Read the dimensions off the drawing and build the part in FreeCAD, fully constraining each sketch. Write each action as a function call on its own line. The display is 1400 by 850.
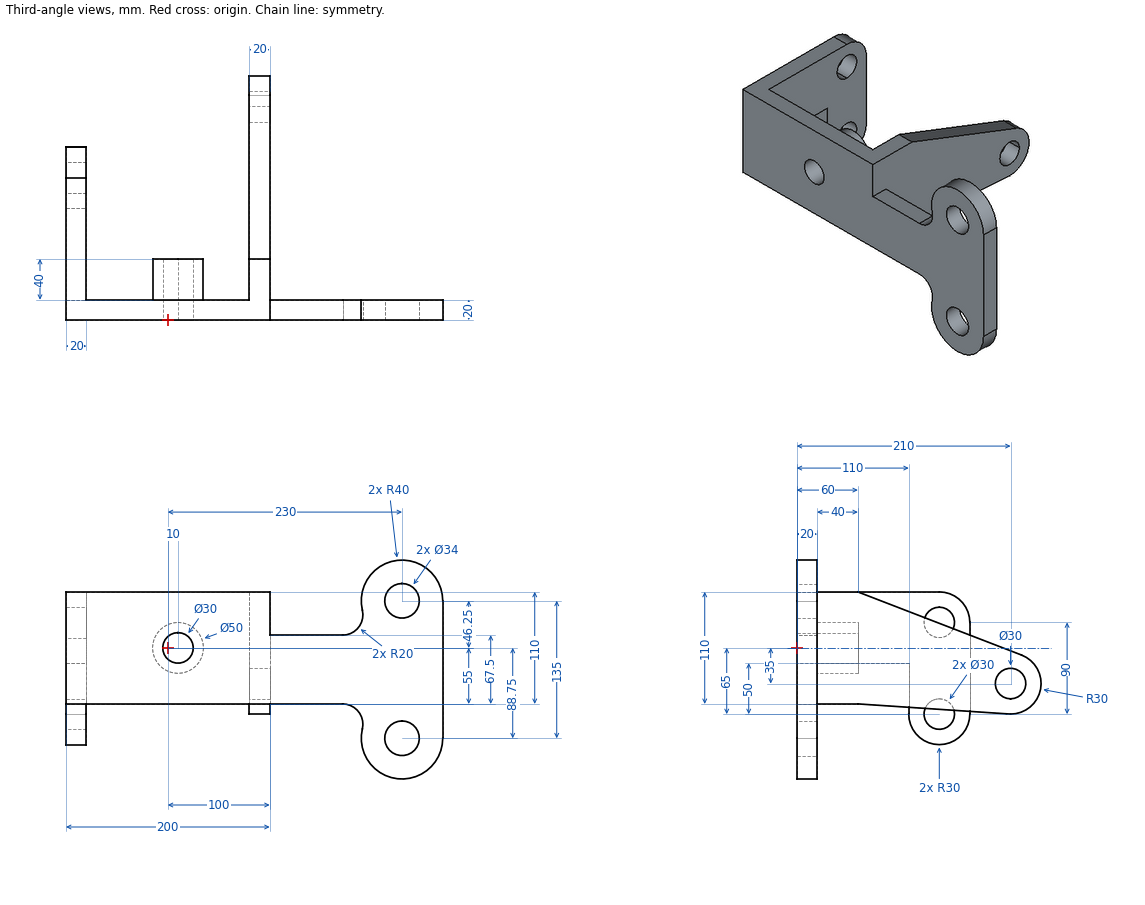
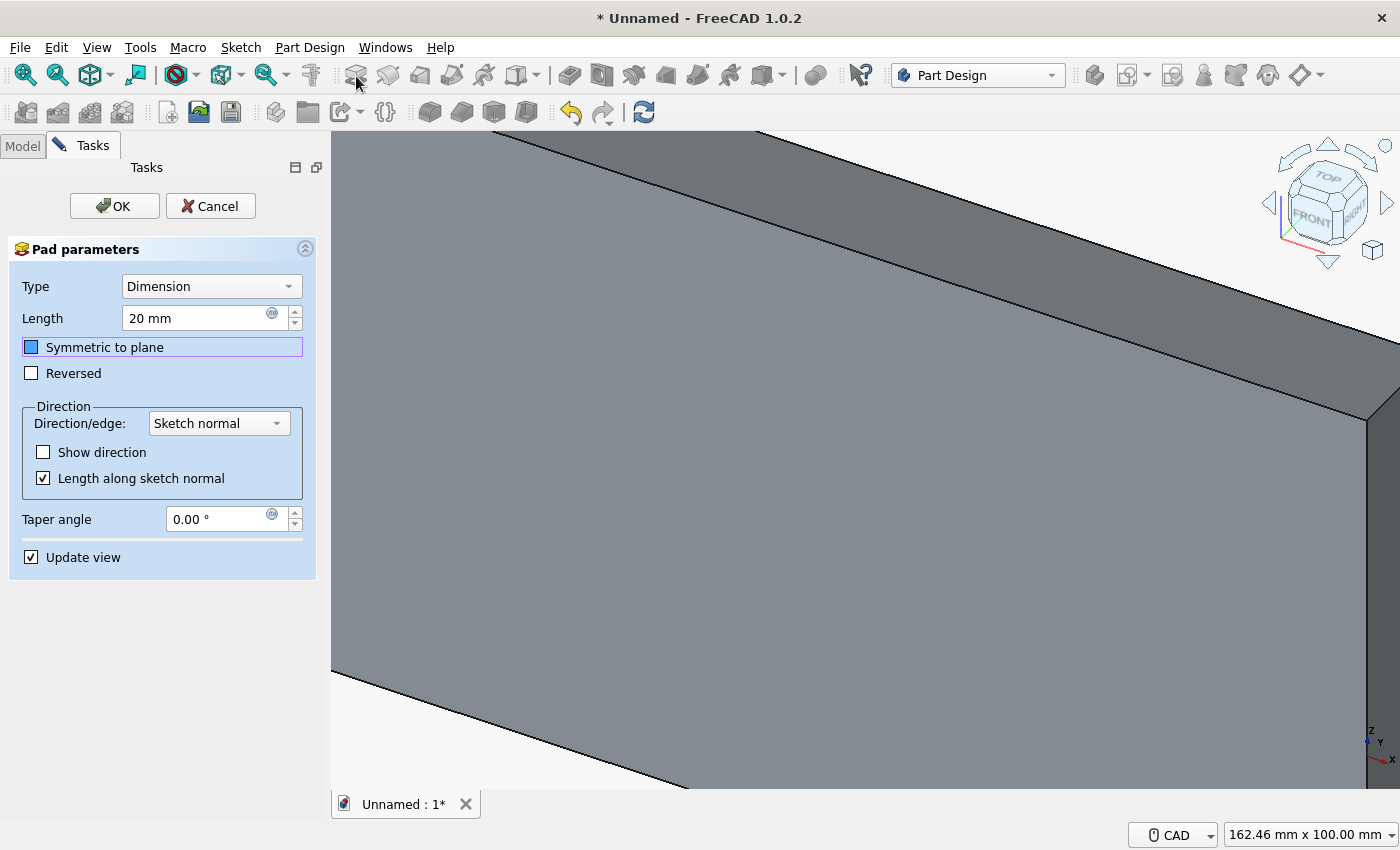
click(30, 373)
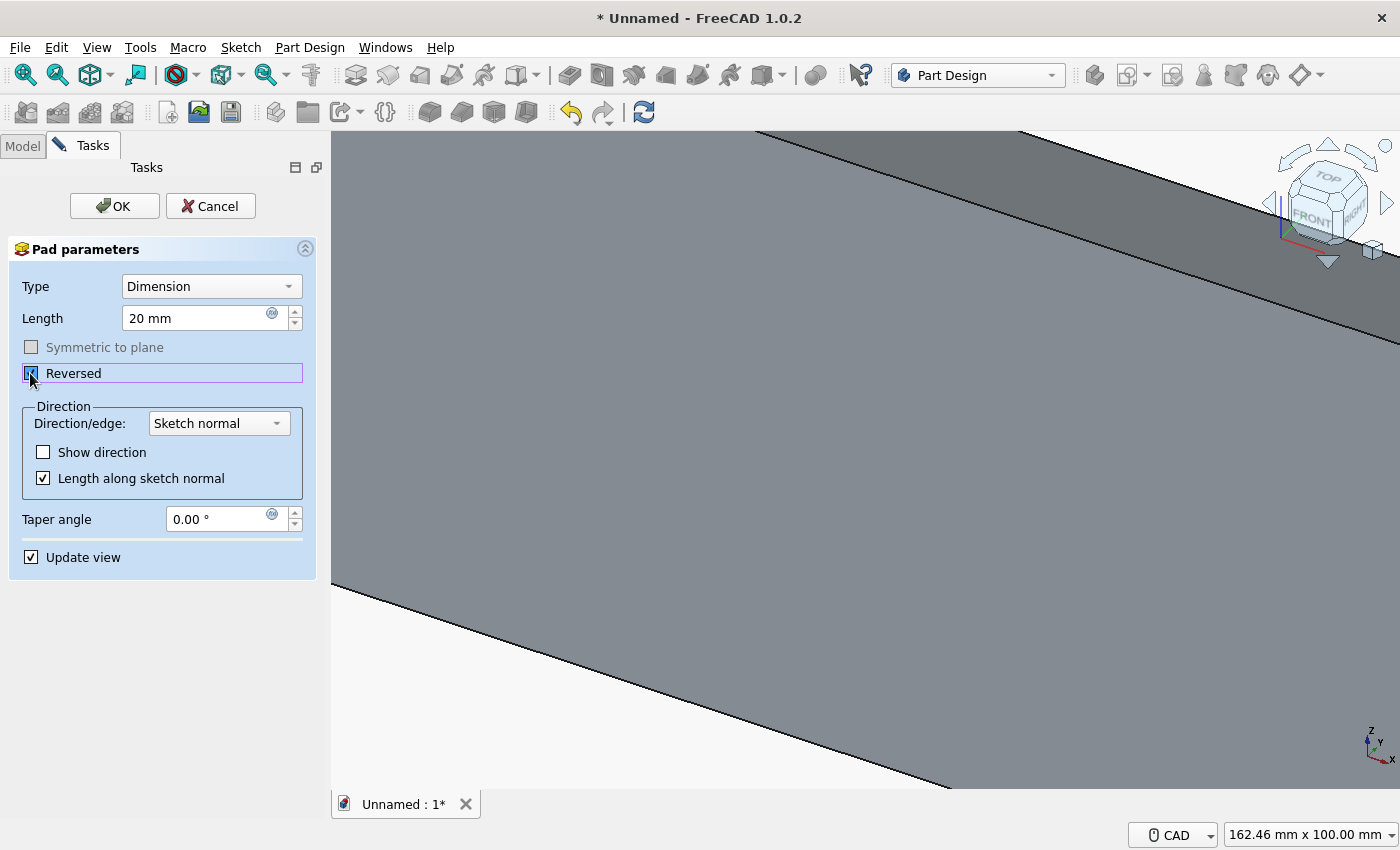
click(115, 206)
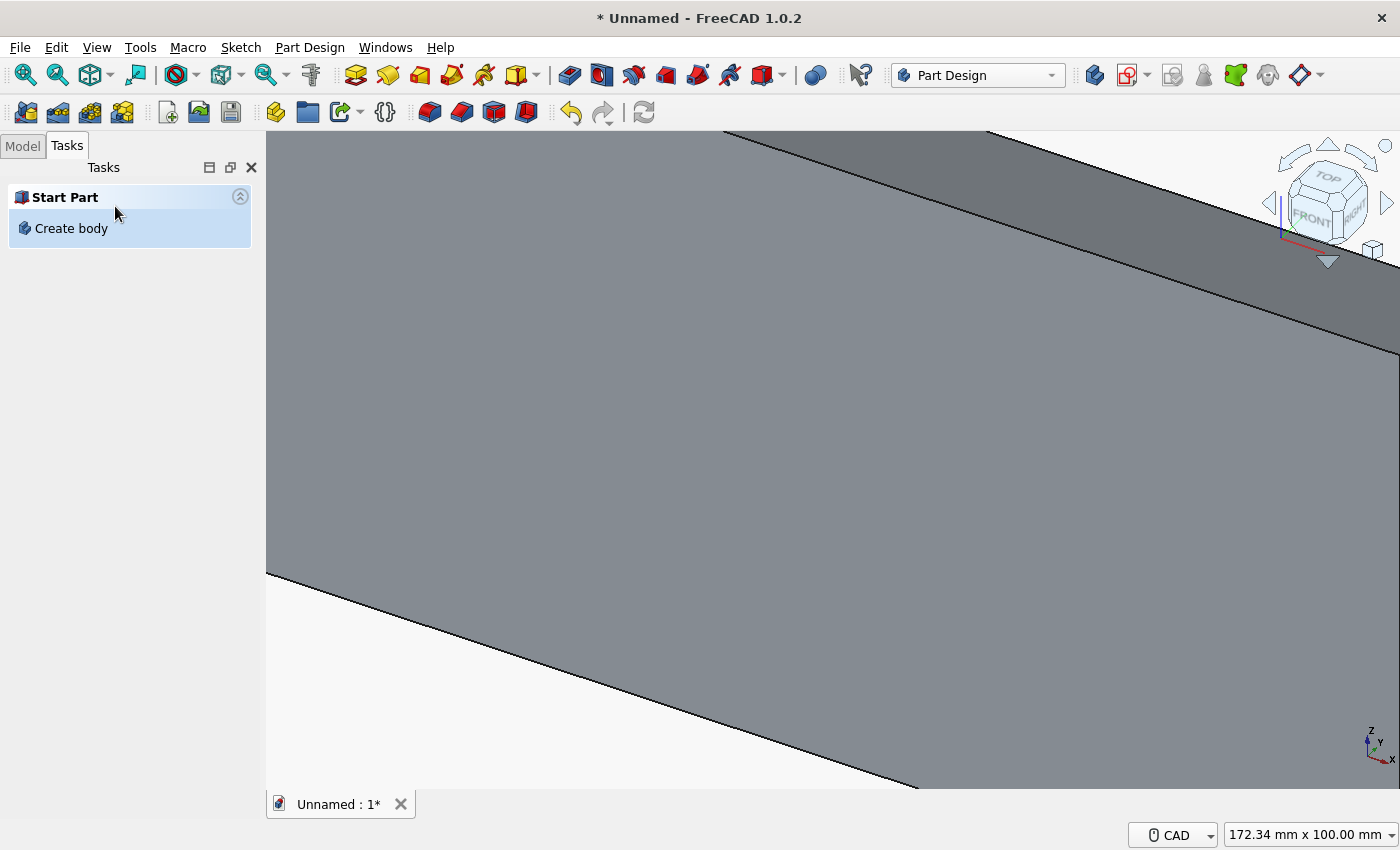
key(v)
key(f)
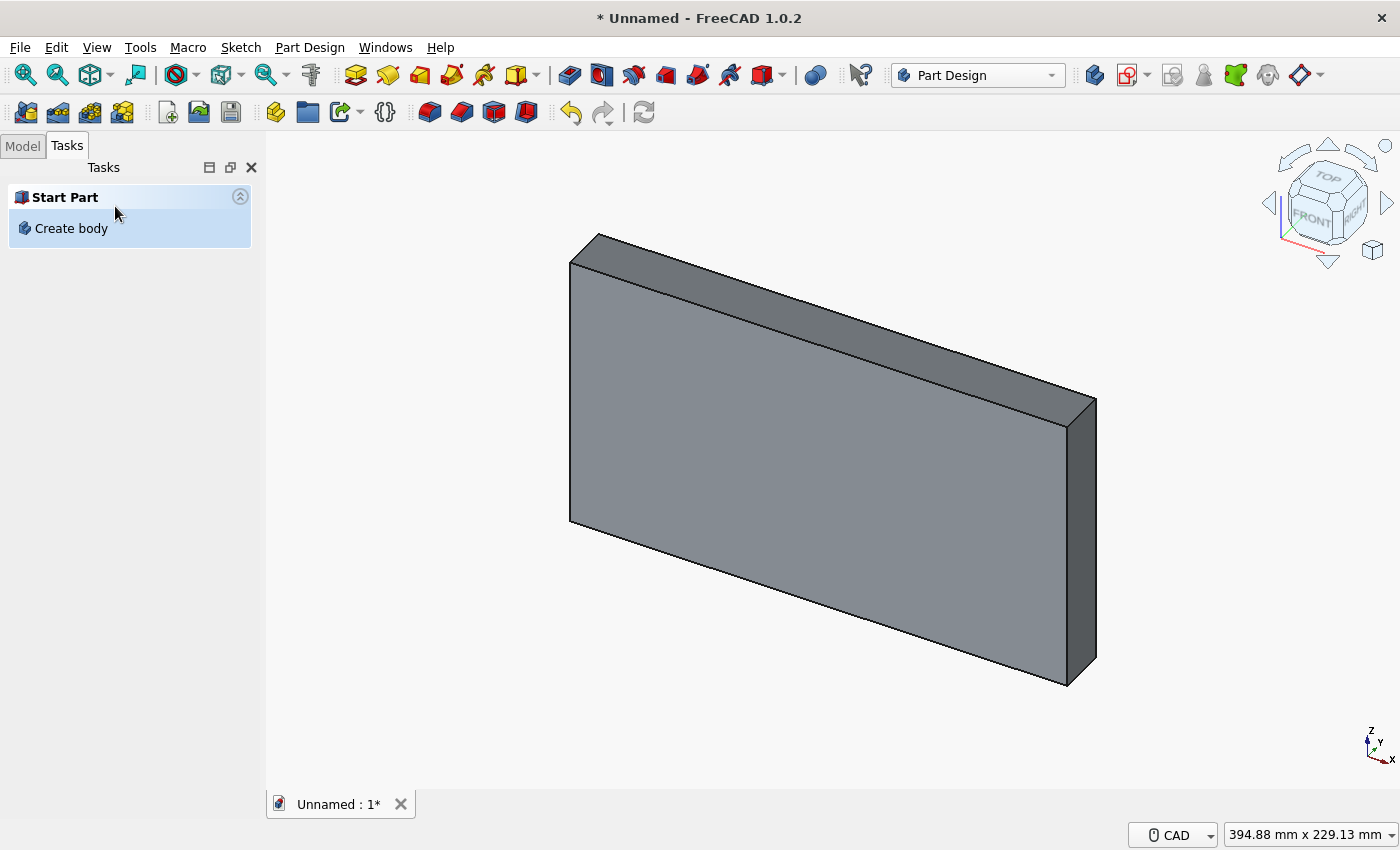
key(4)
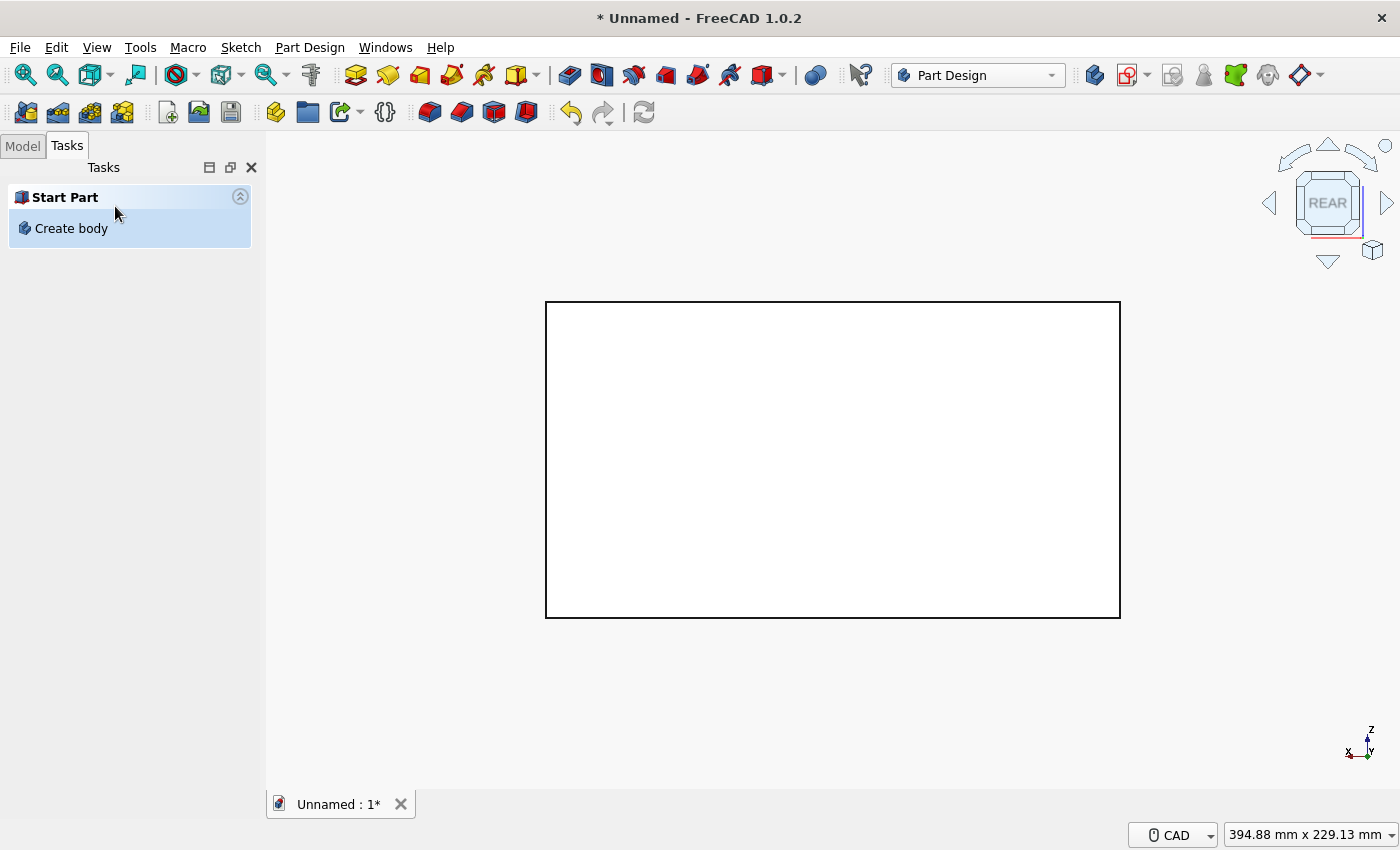
click(751, 459)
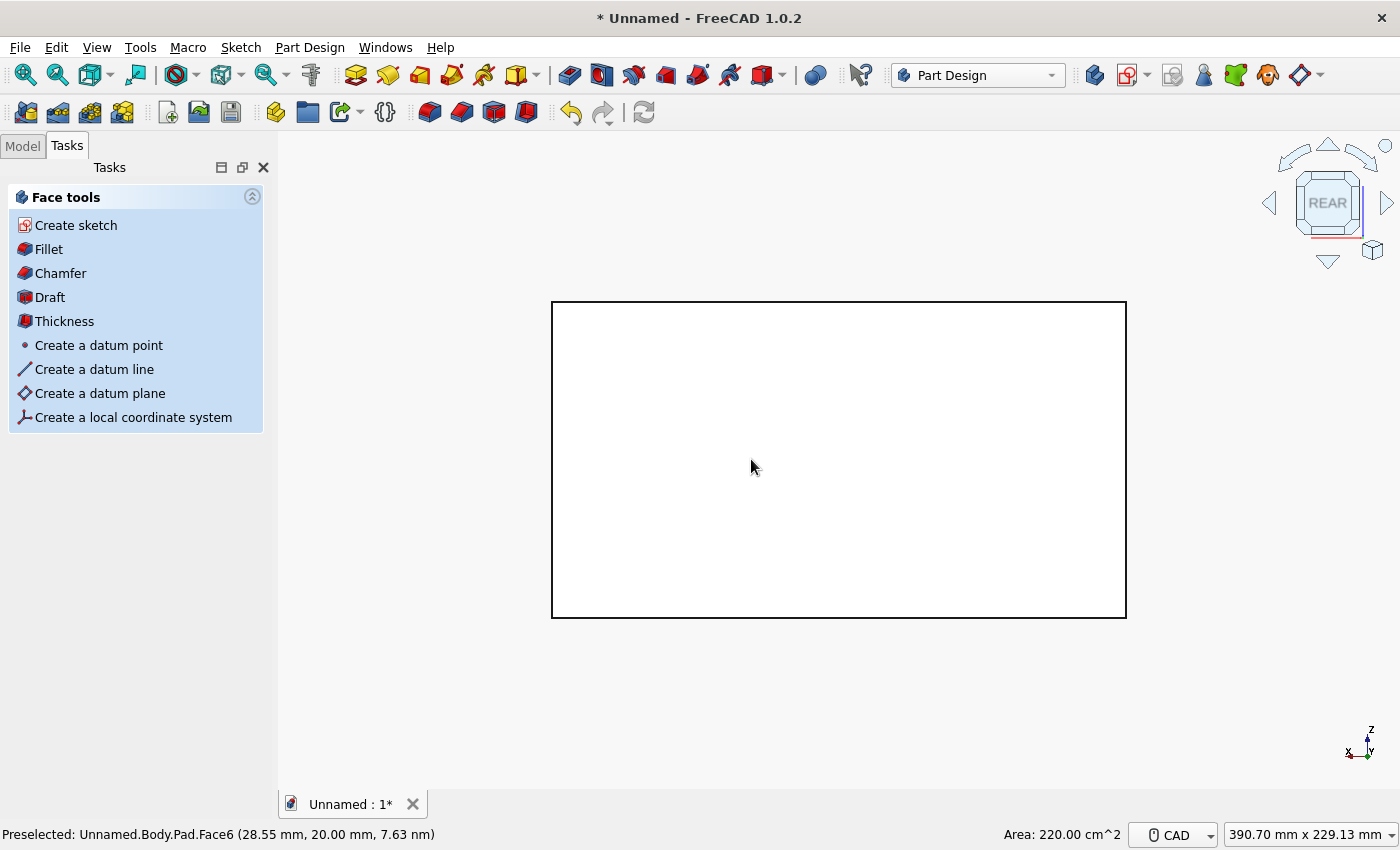
click(1128, 76)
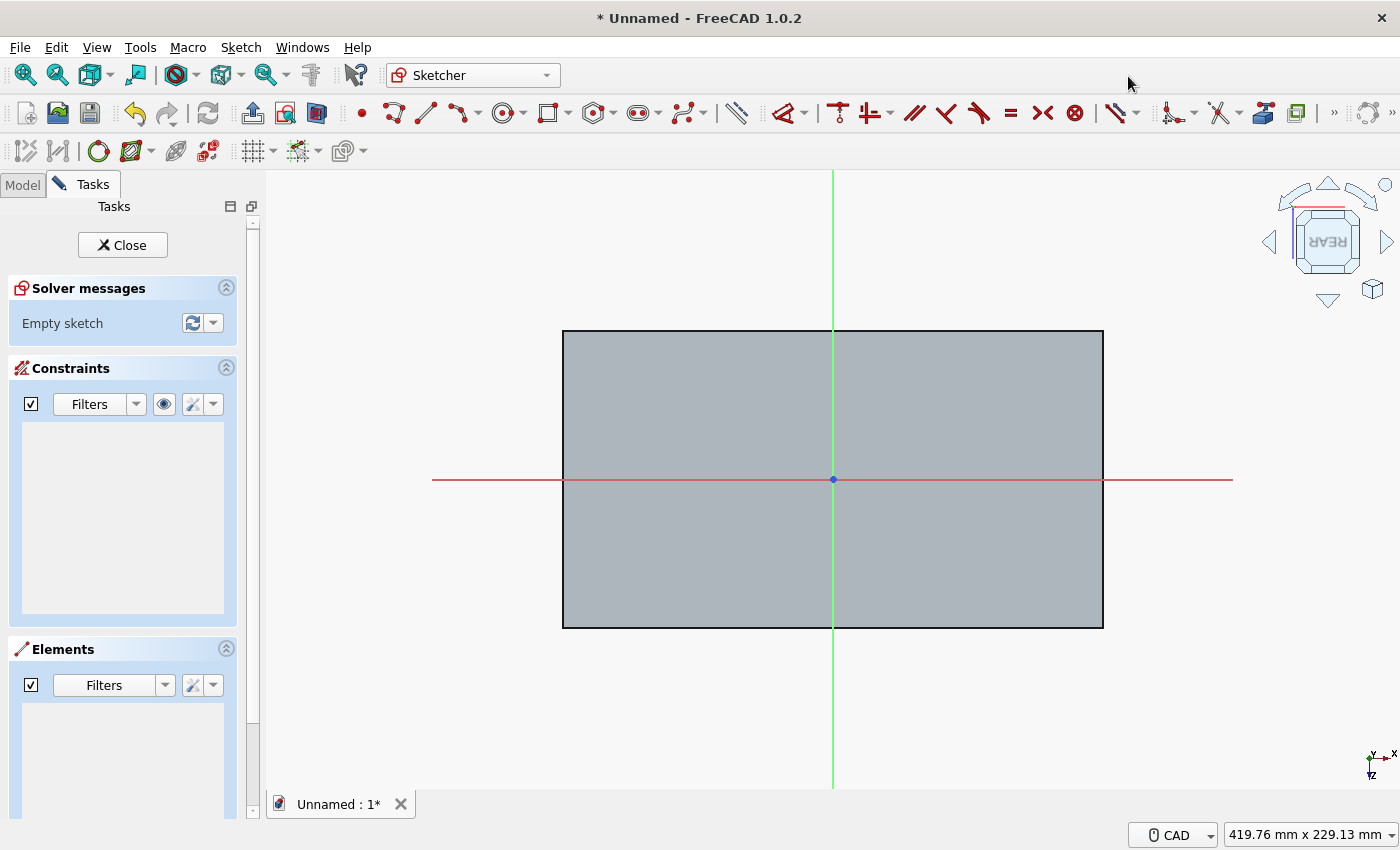
scroll(294, 596, down, 2)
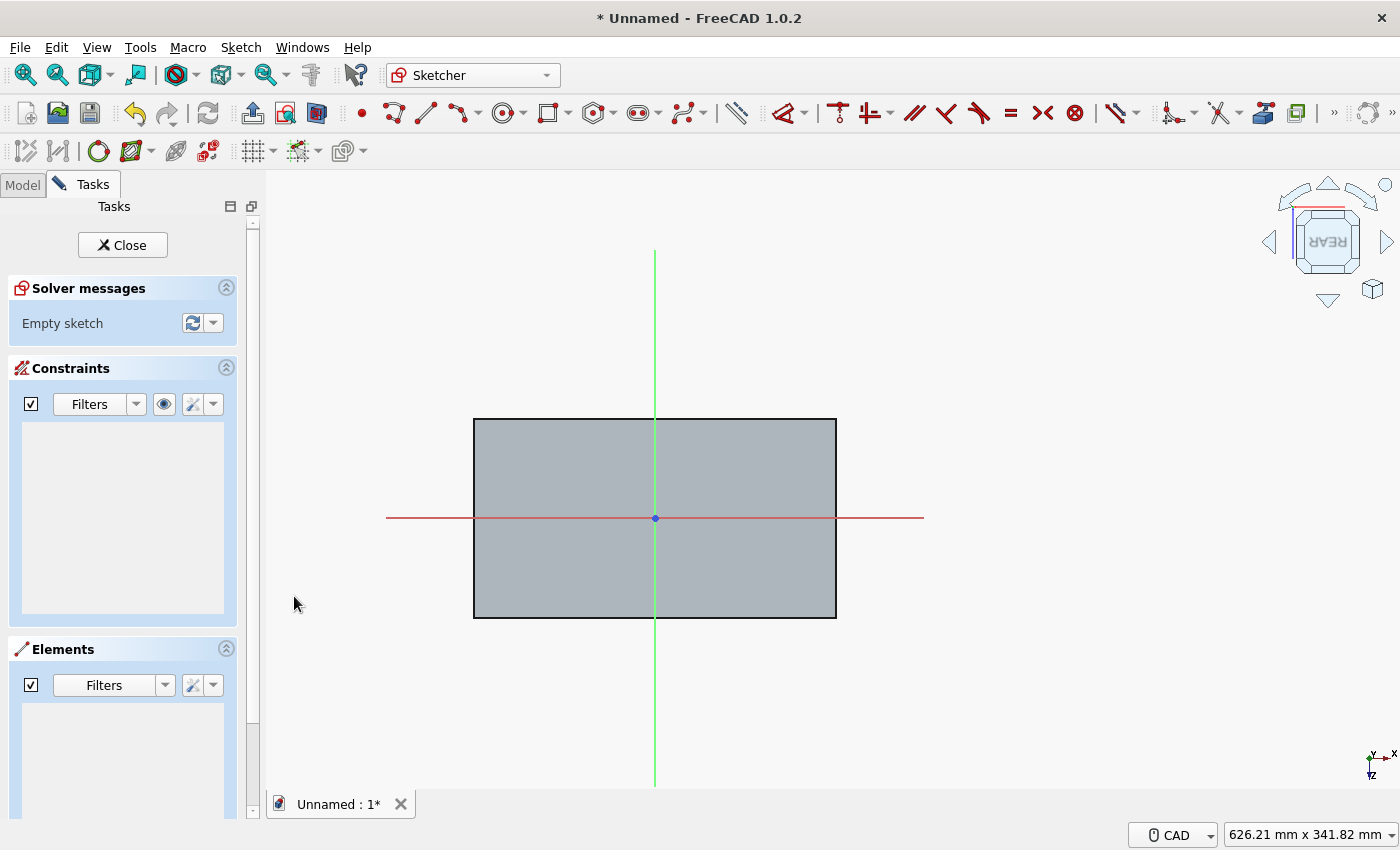
key(g)
key(l)